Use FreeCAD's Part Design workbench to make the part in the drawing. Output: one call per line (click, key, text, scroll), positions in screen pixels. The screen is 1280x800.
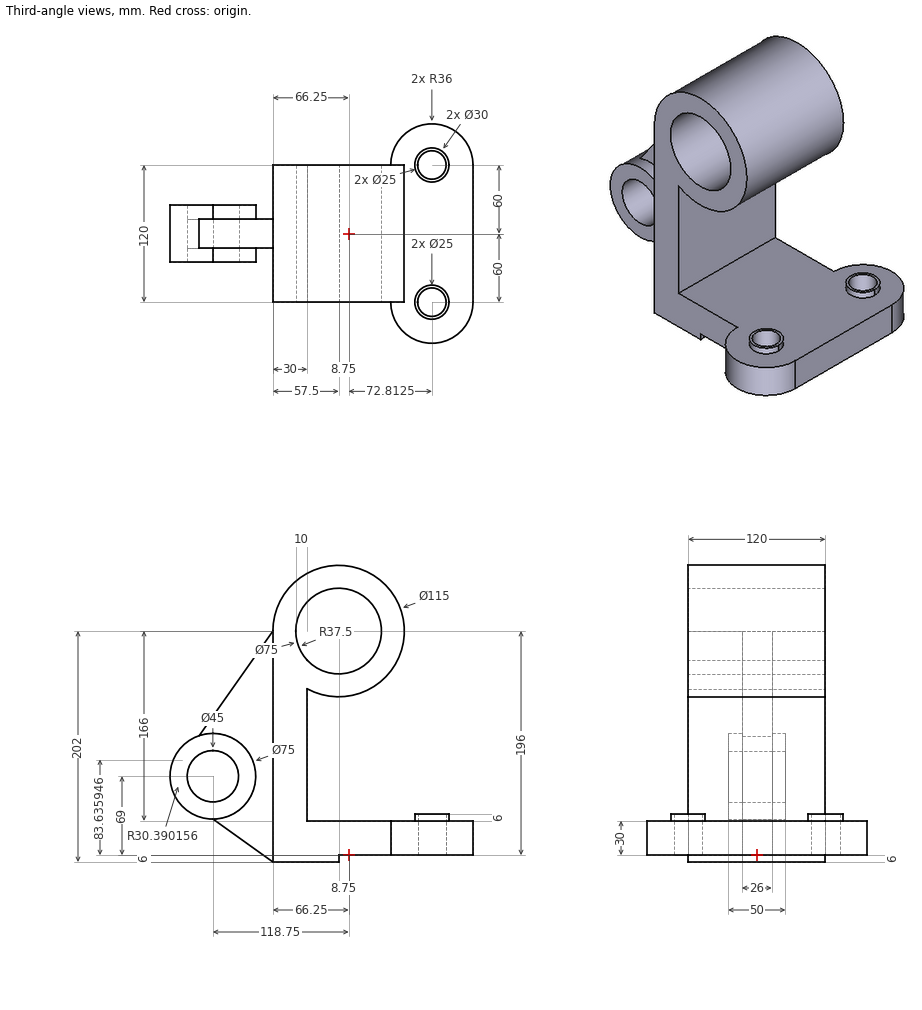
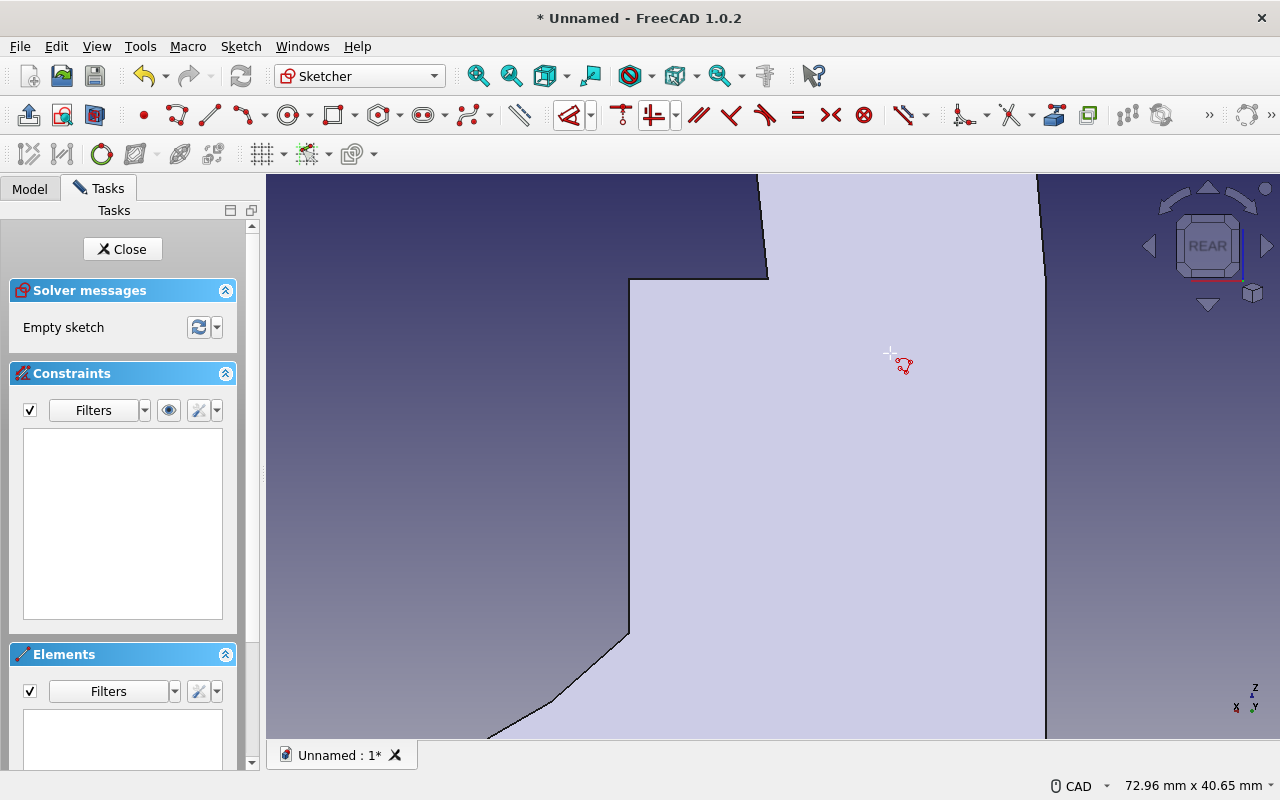
click(768, 279)
click(629, 279)
click(629, 633)
right_click(629, 633)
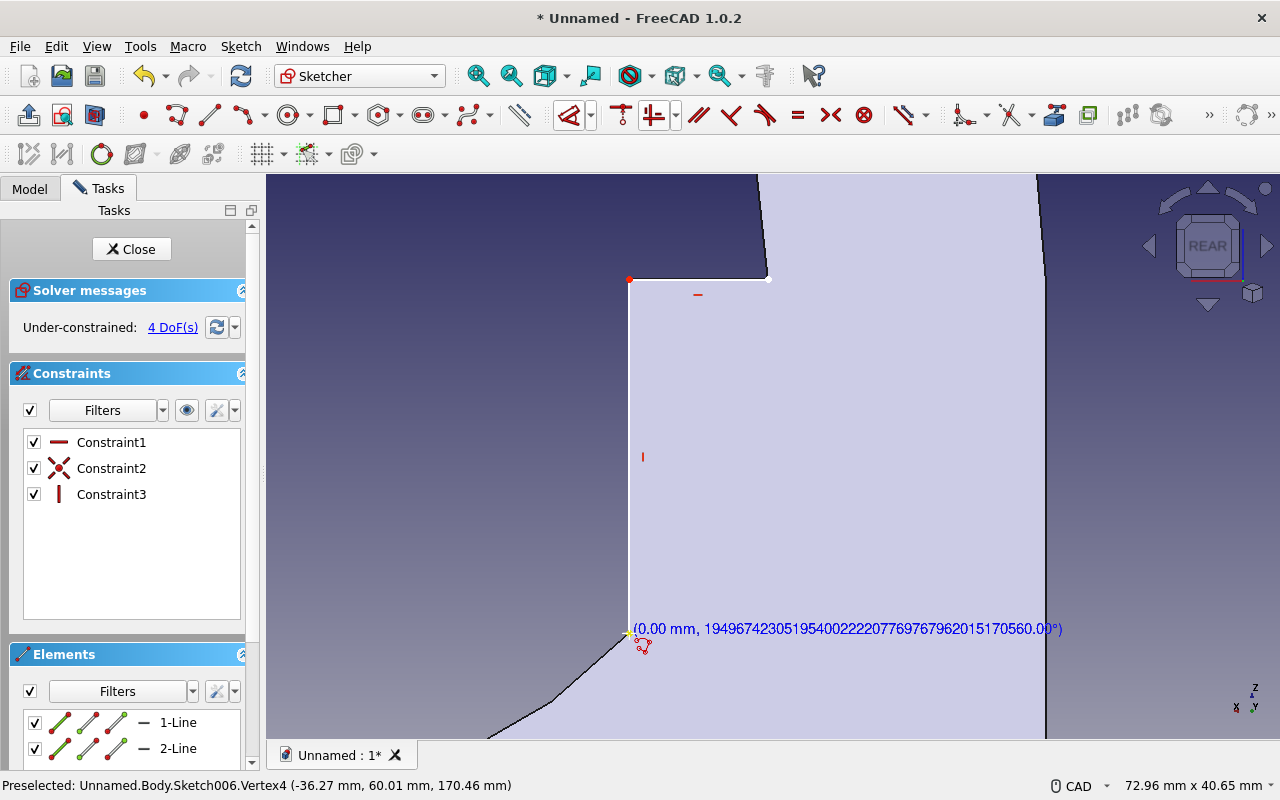
click(242, 116)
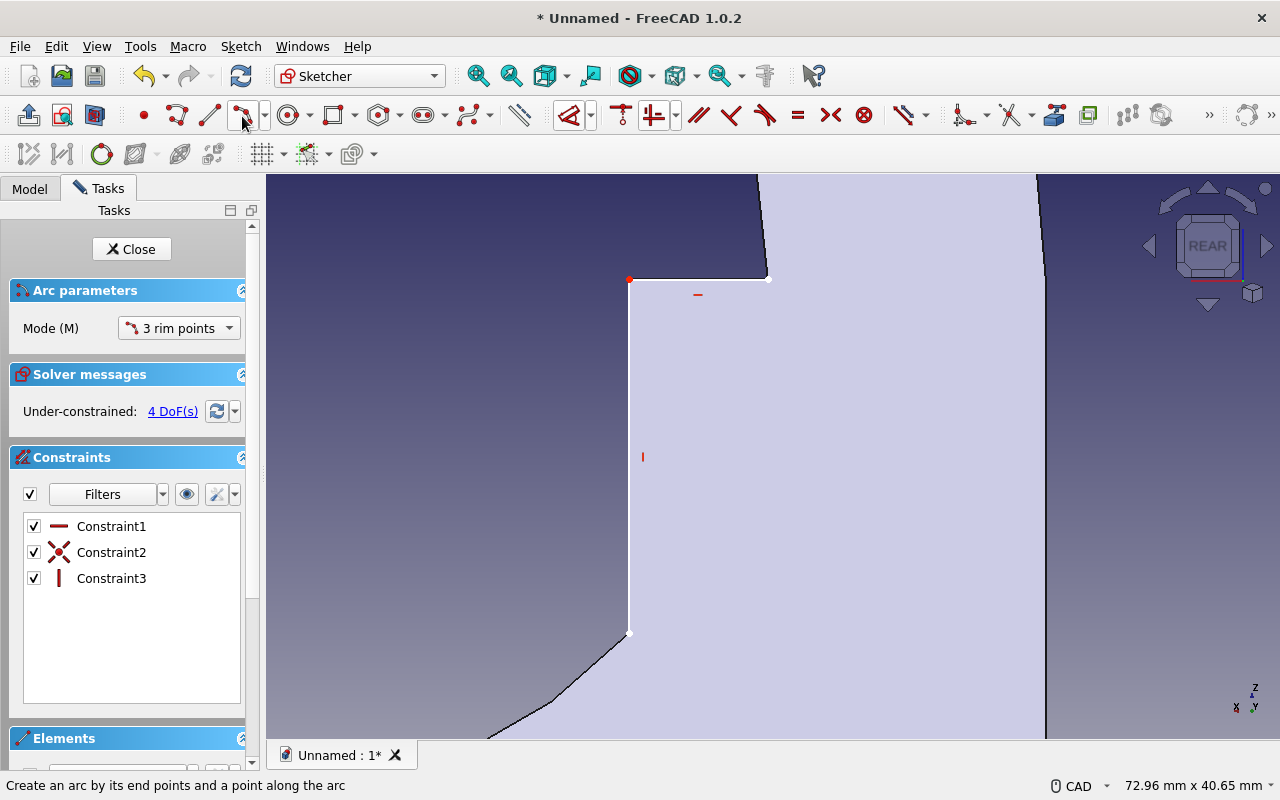
click(629, 634)
click(768, 280)
click(732, 469)
key(Escape)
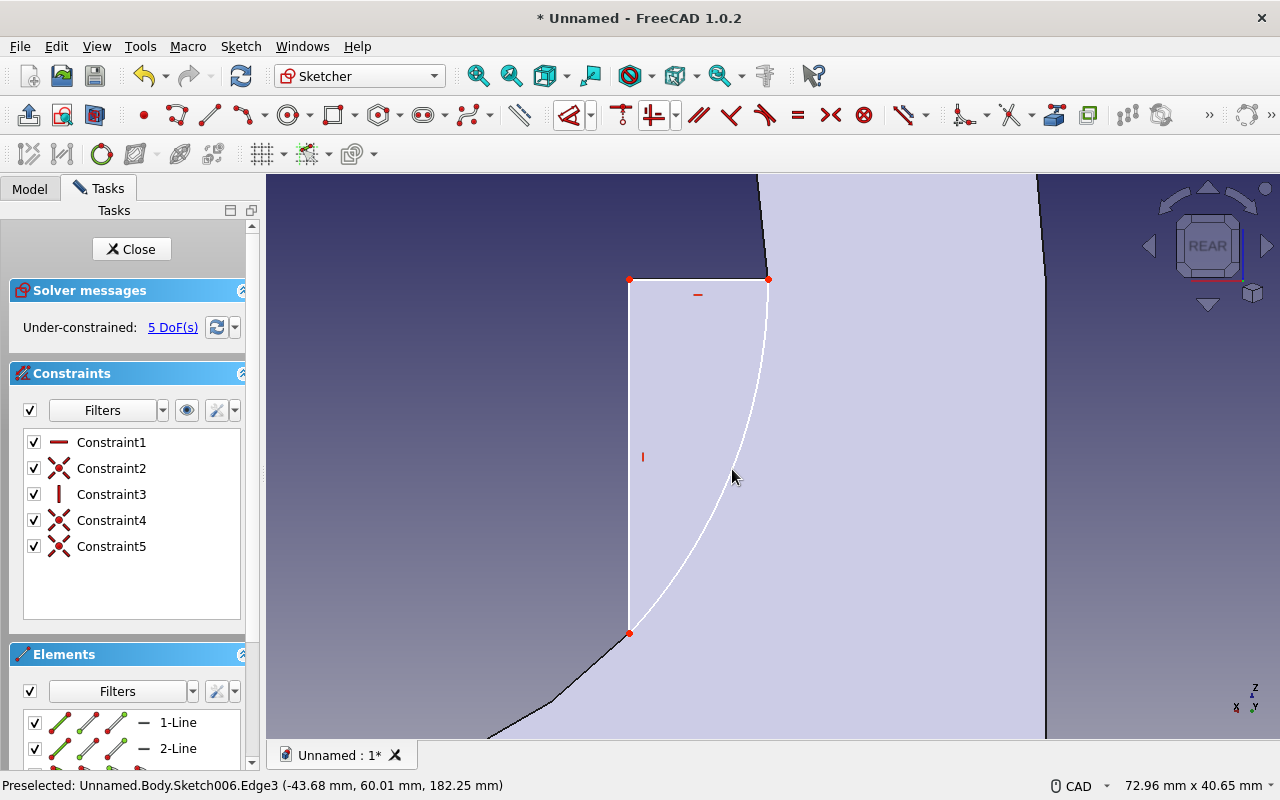
click(698, 540)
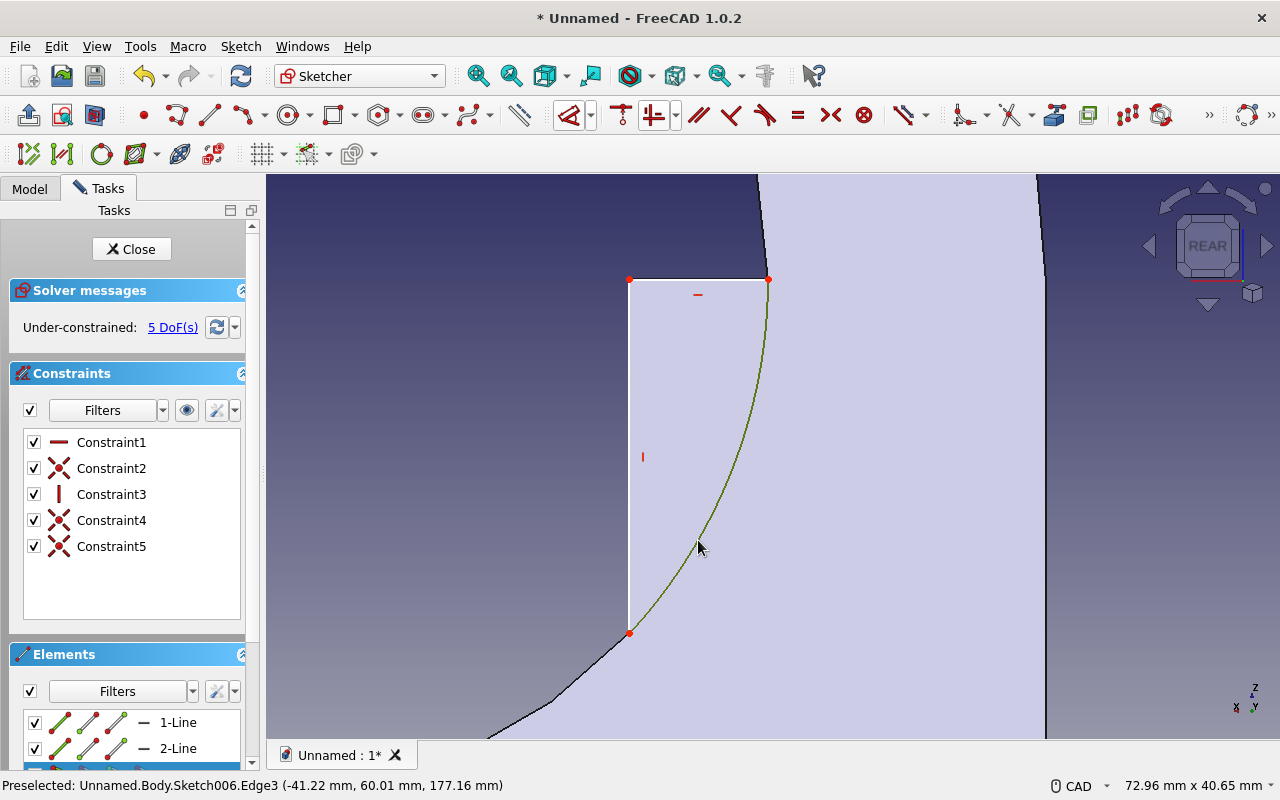
key(k)
key(r)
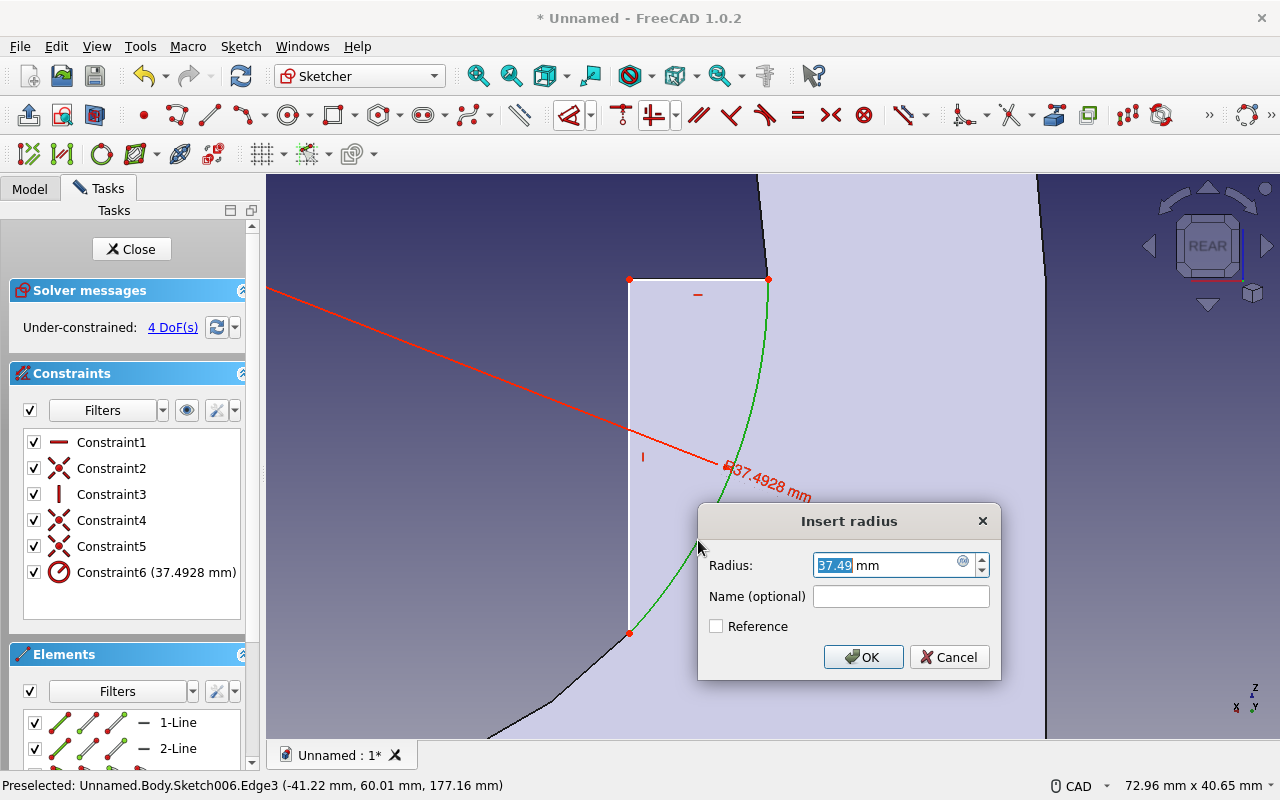
text(37.5)
key(Return)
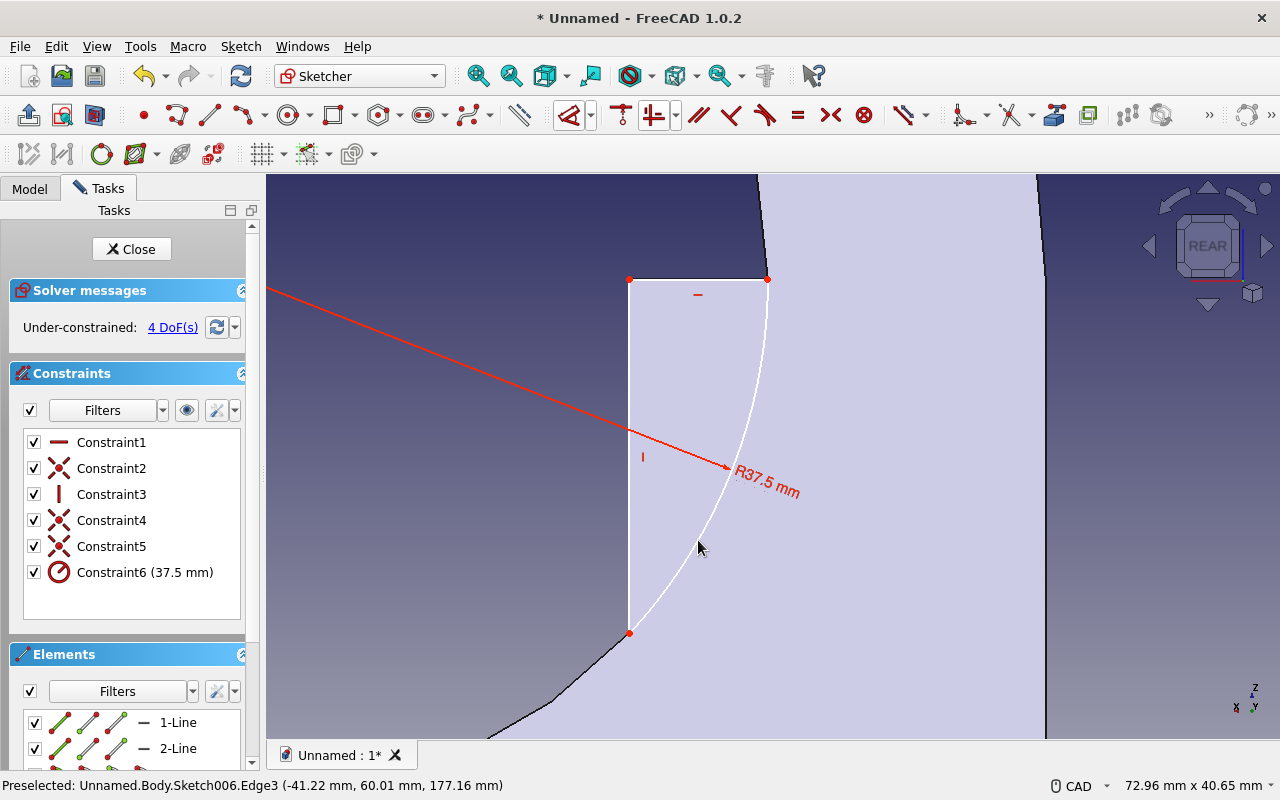
click(726, 280)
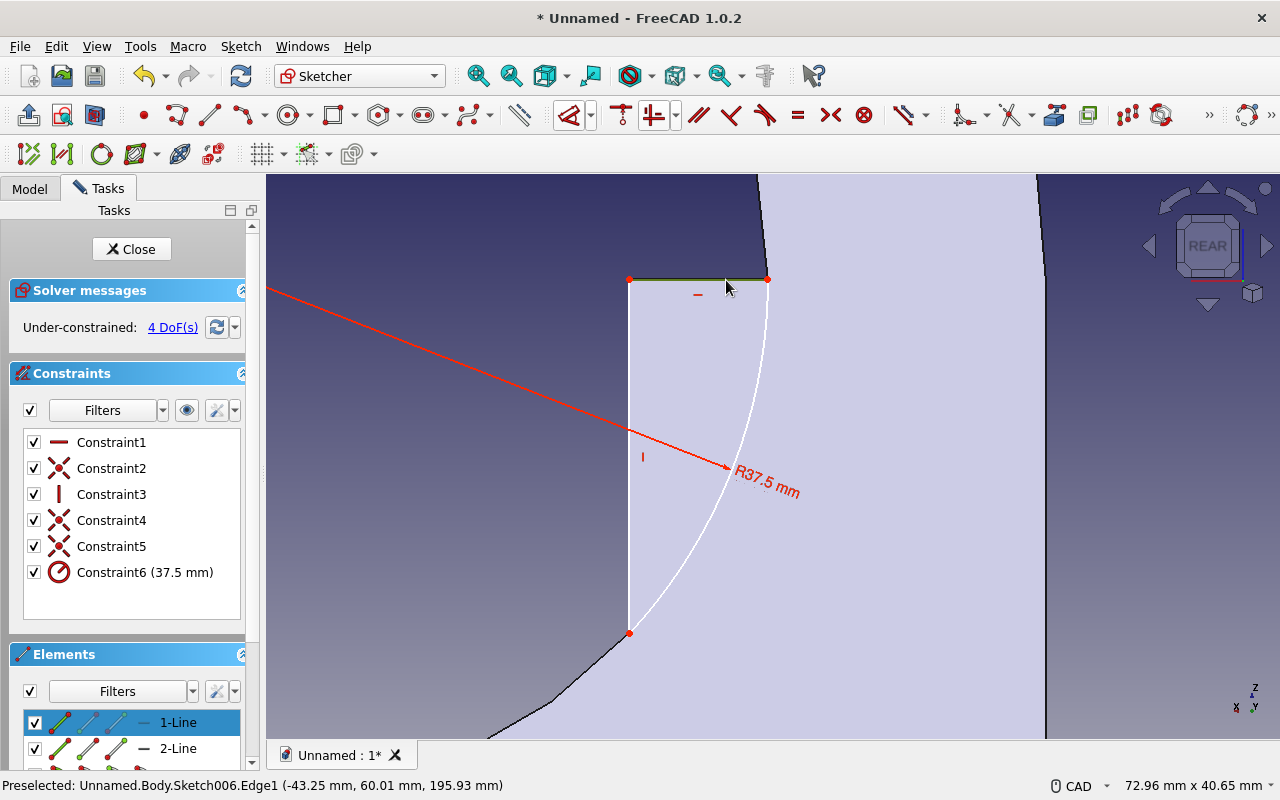
key(l)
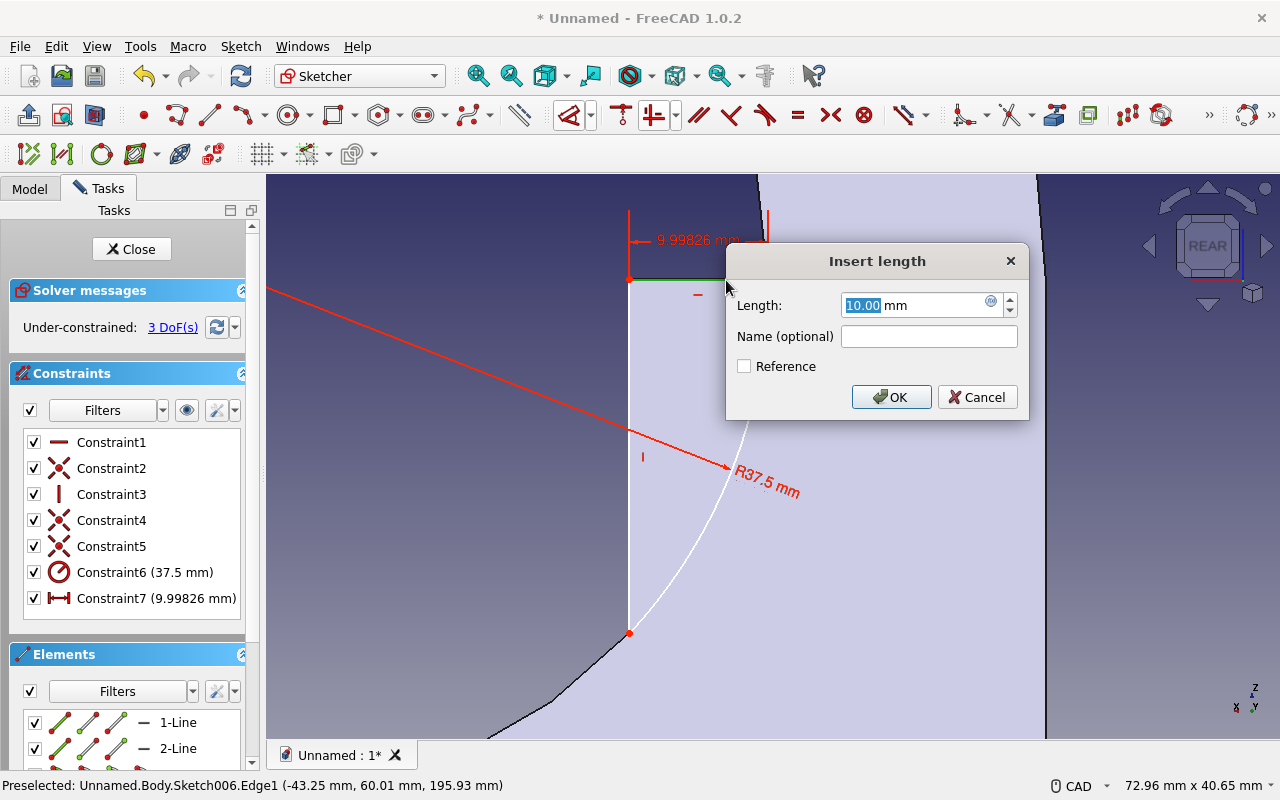
text(10)
key(Return)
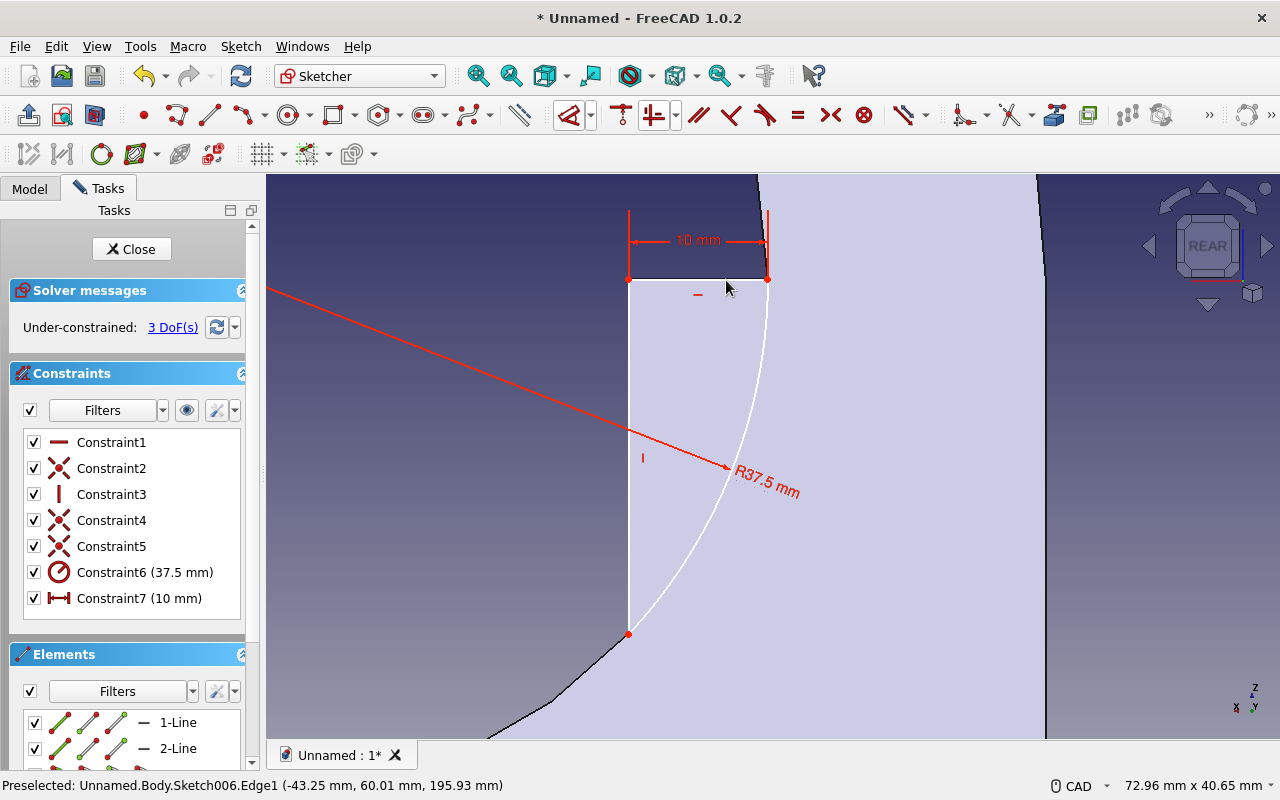
click(768, 280)